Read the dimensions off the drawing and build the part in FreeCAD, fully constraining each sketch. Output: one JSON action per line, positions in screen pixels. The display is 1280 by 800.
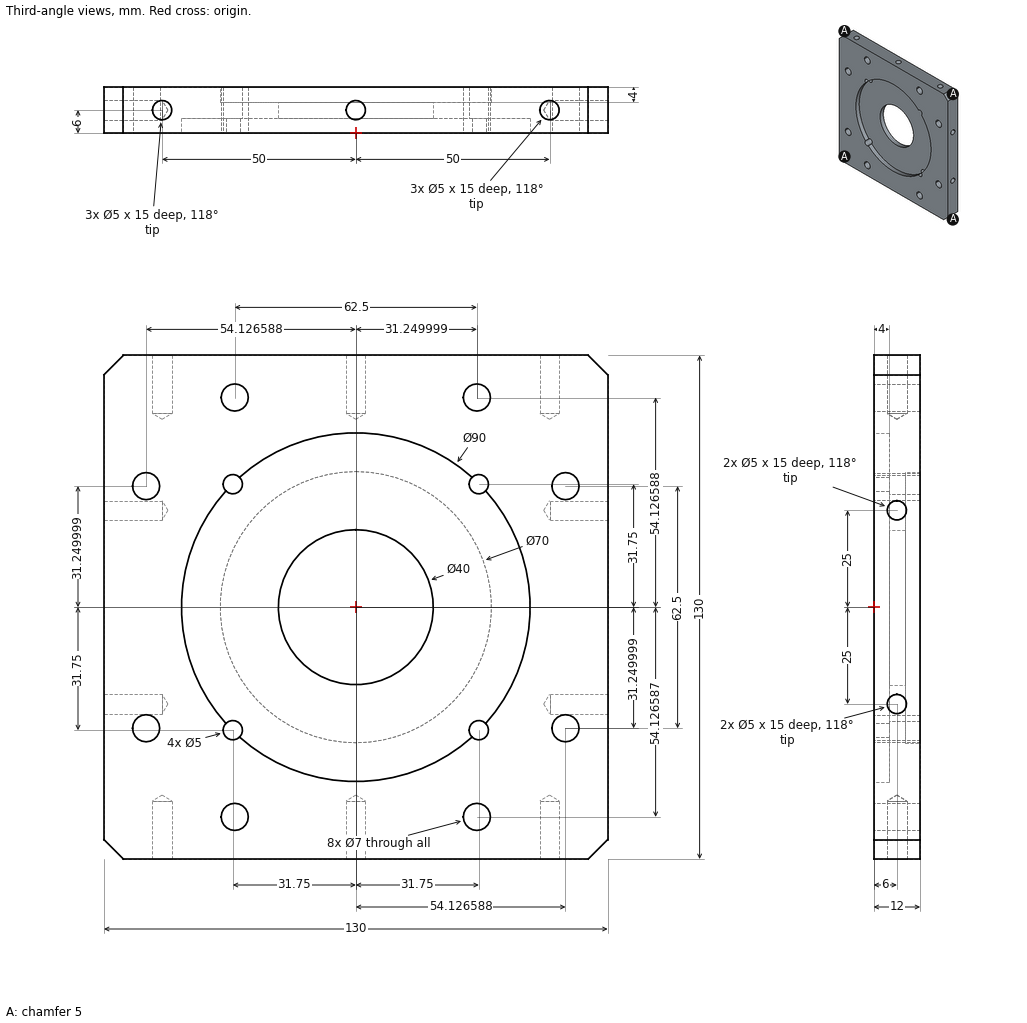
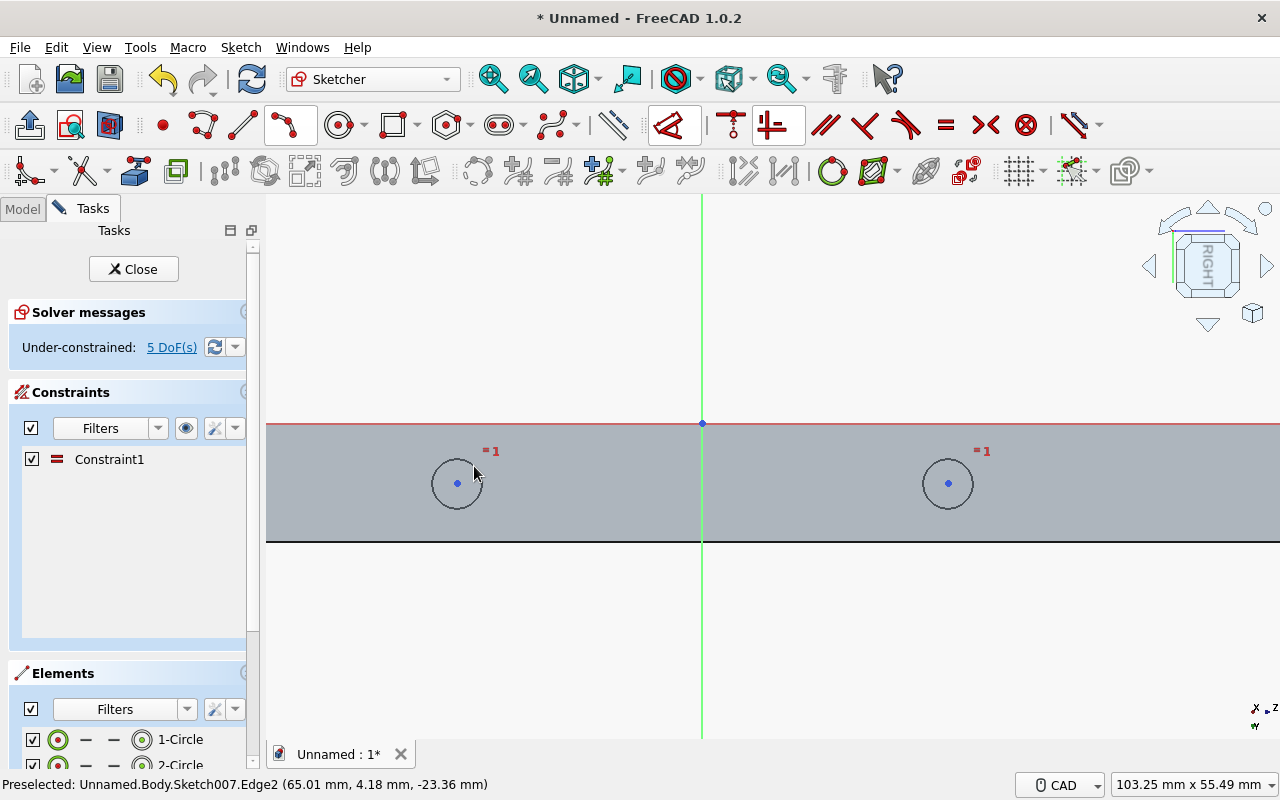
{"action": "left_click", "coordinate": [948, 484]}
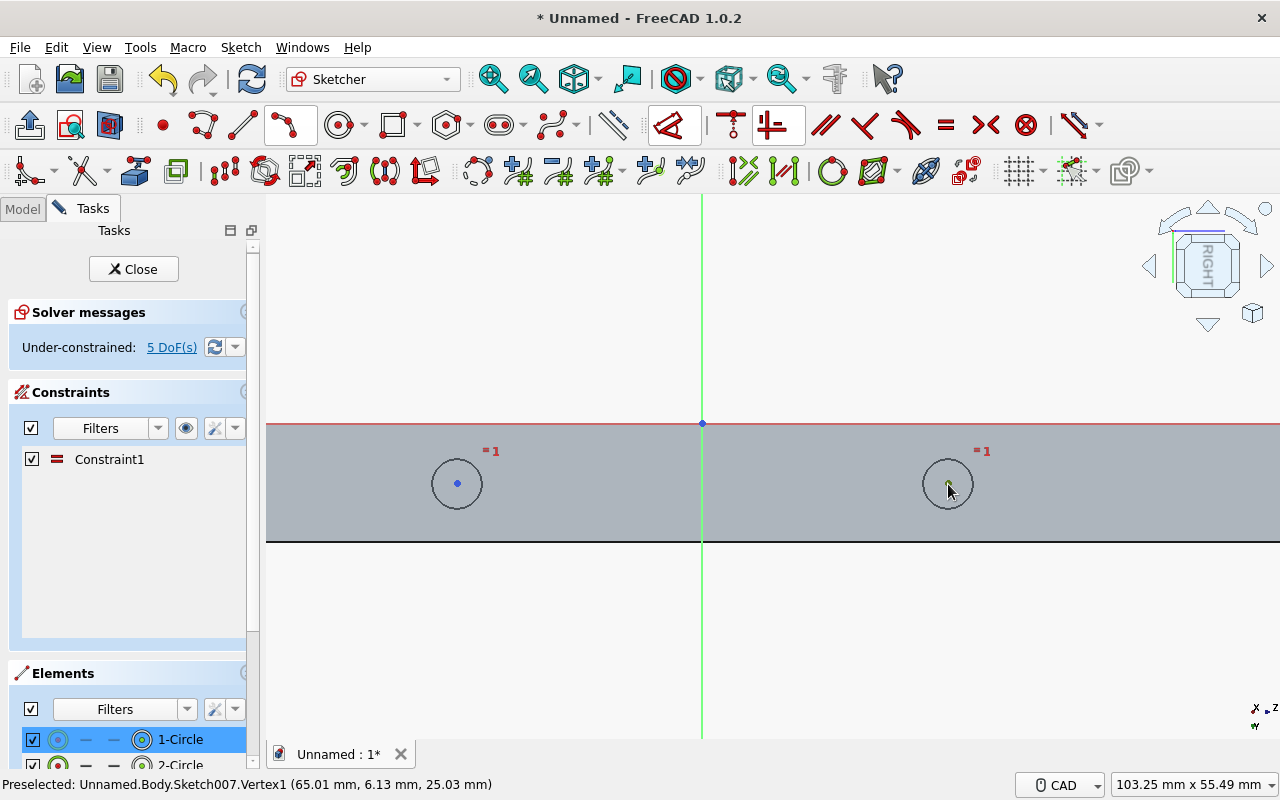
{"action": "left_click", "coordinate": [457, 484]}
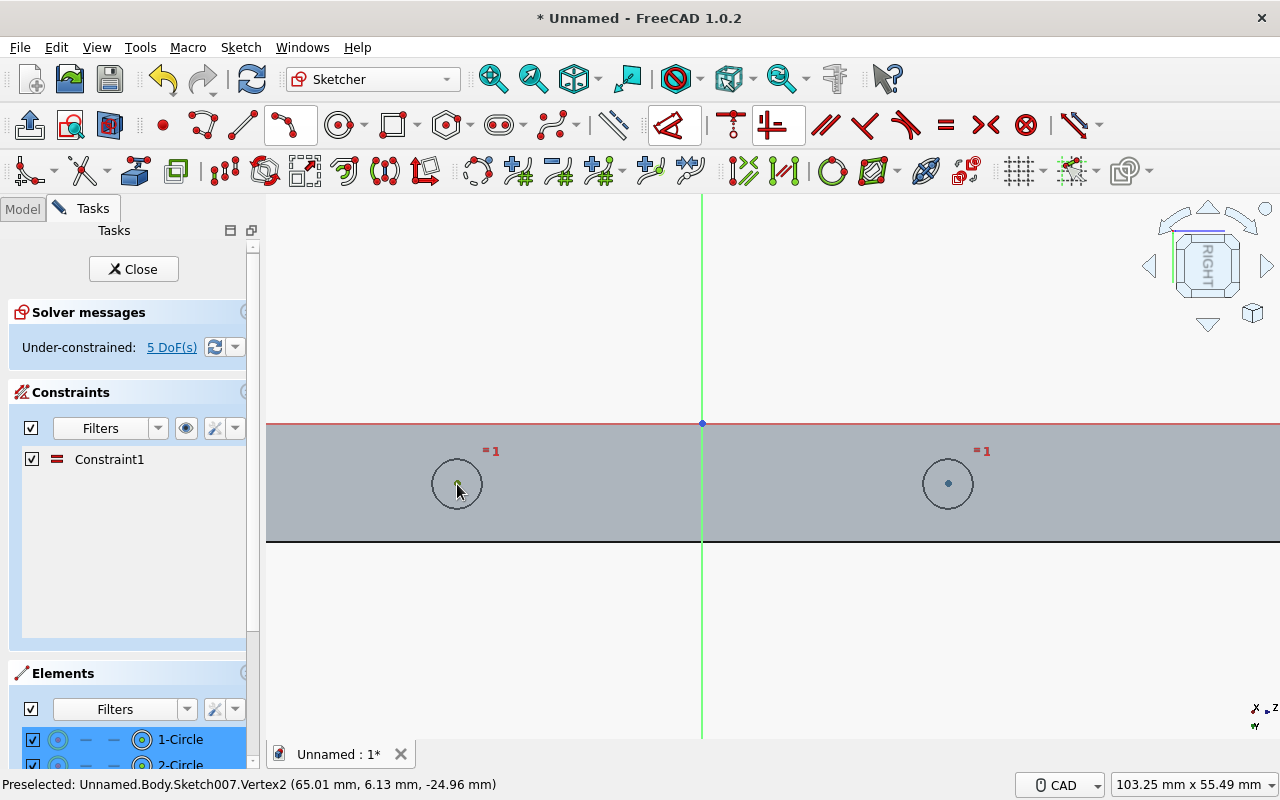
{"action": "left_click", "coordinate": [800, 126]}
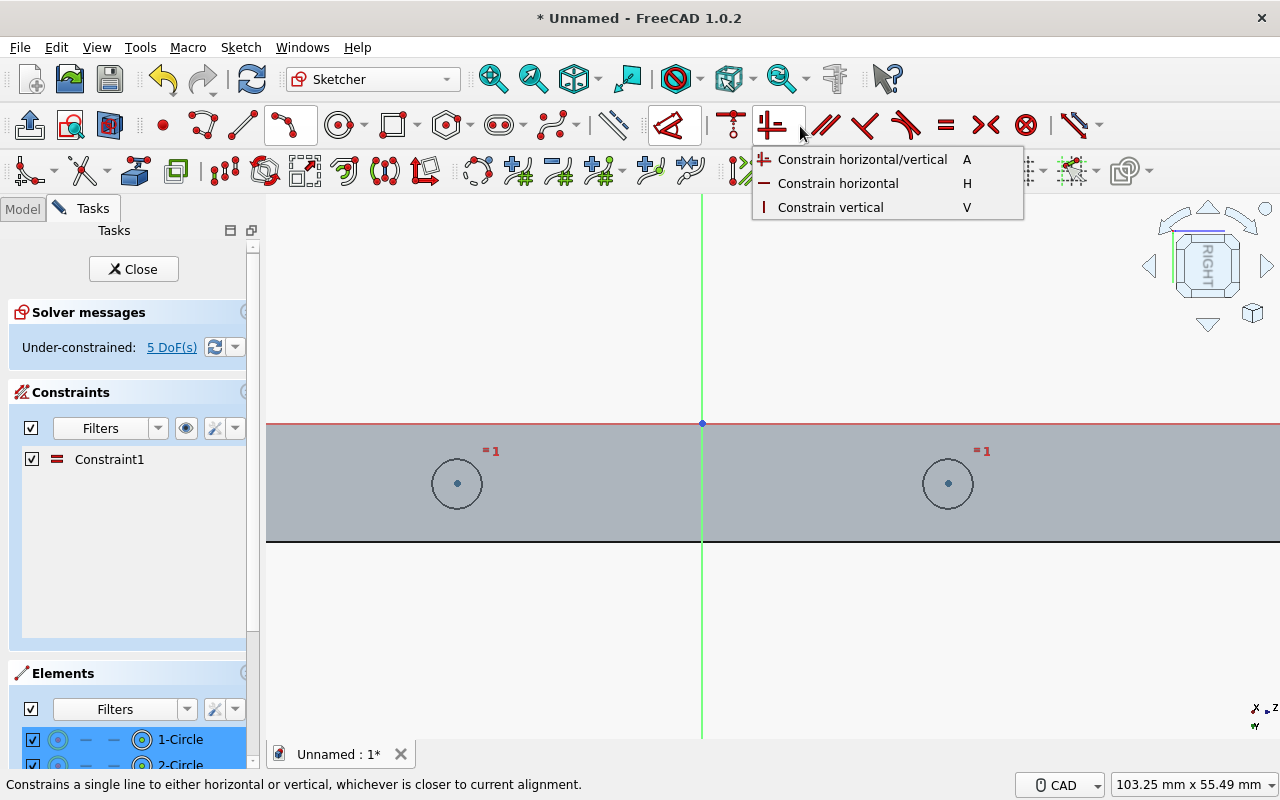
{"action": "left_click", "coordinate": [888, 183]}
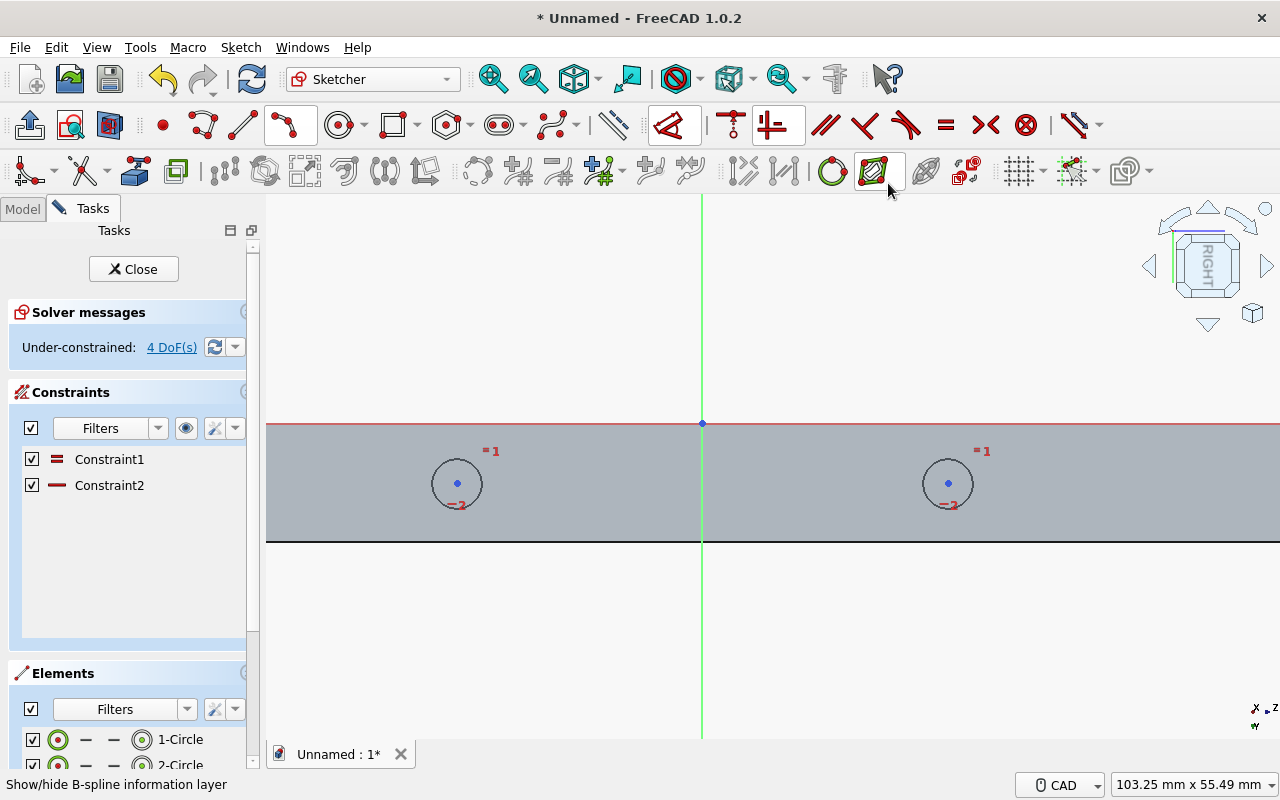
{"action": "left_click", "coordinate": [668, 126]}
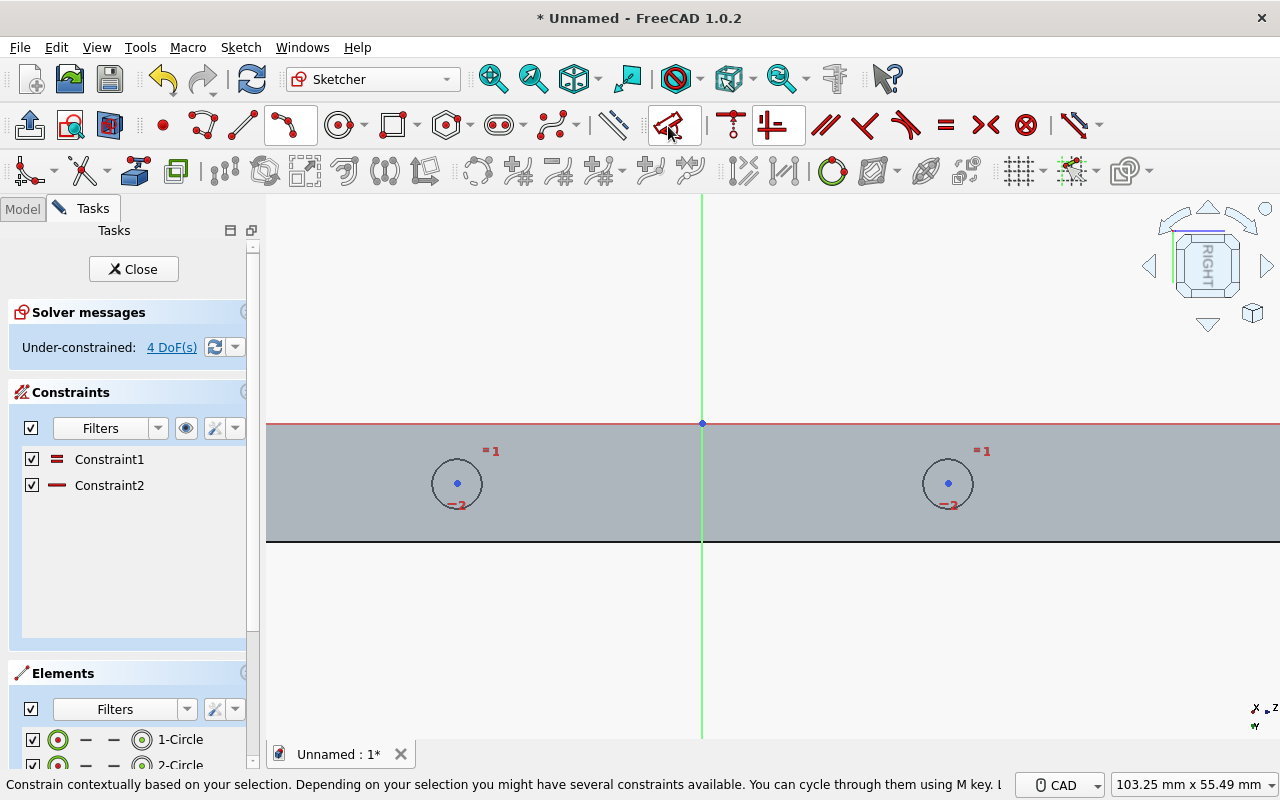
{"action": "left_click", "coordinate": [965, 466]}
{"action": "left_click", "coordinate": [987, 443]}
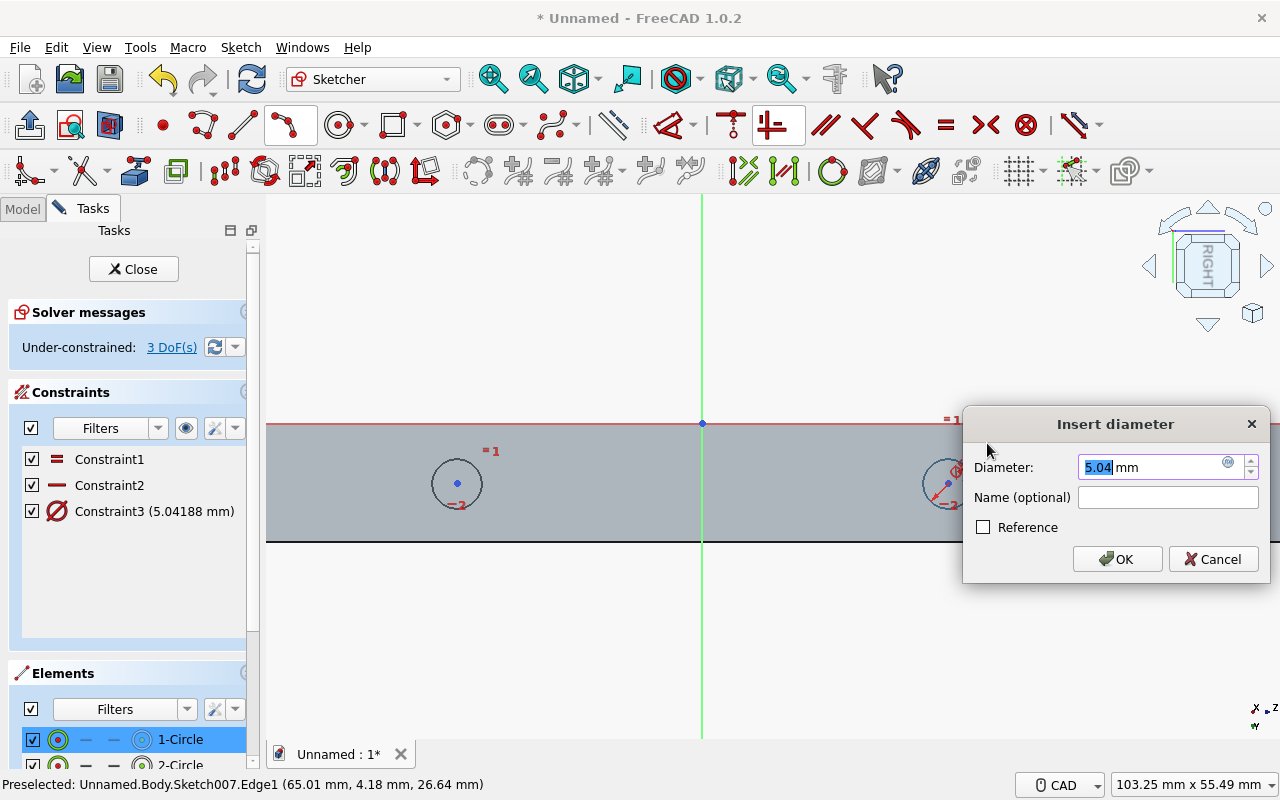
{"action": "type", "text": "5"}
{"action": "key", "text": "Return"}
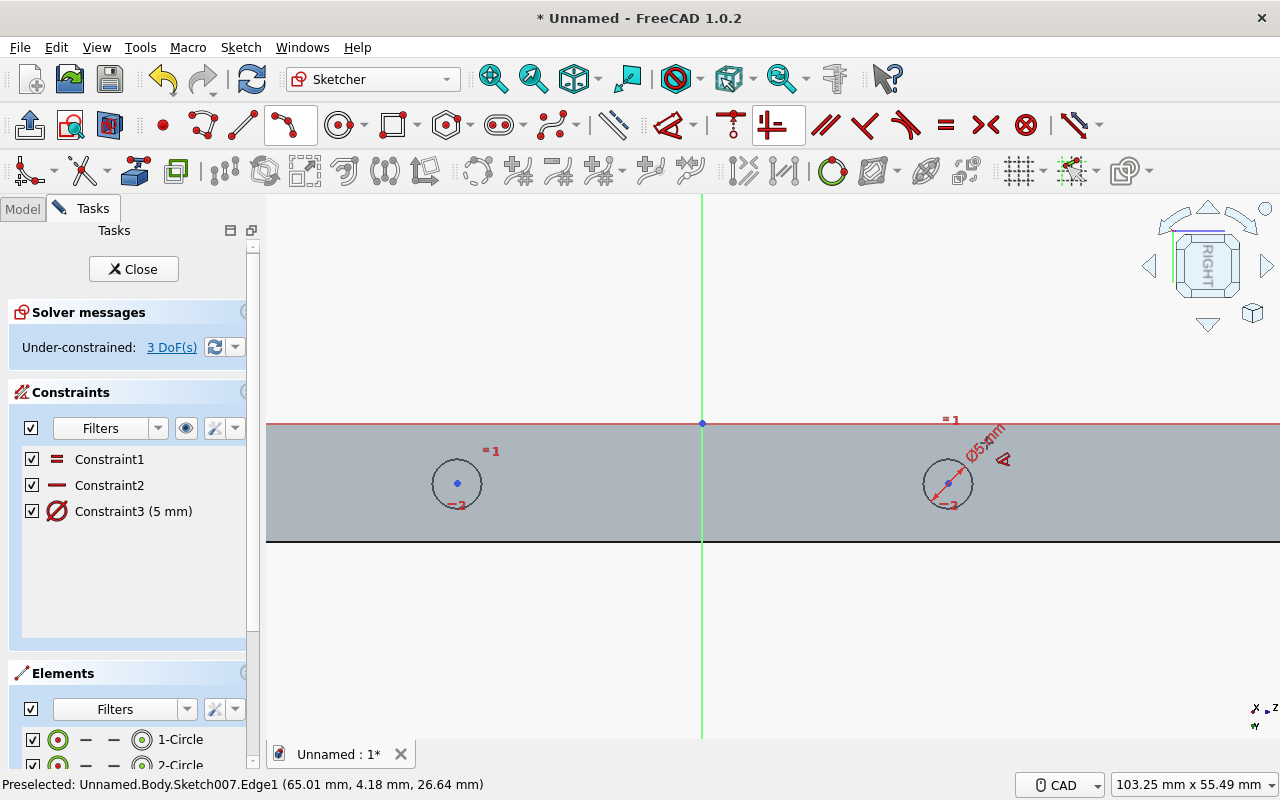
{"action": "left_click", "coordinate": [948, 484]}
{"action": "left_click", "coordinate": [982, 468]}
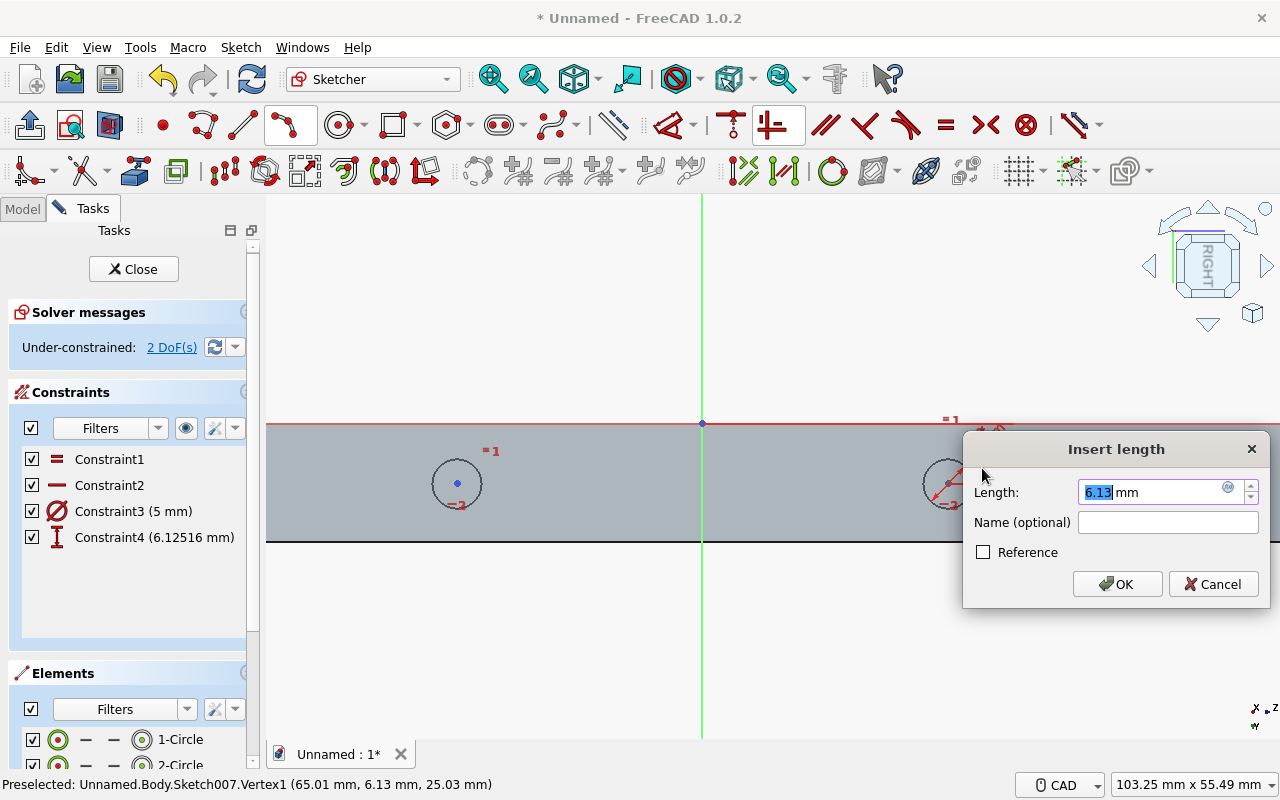
{"action": "type", "text": "6"}
{"action": "key", "text": "Return"}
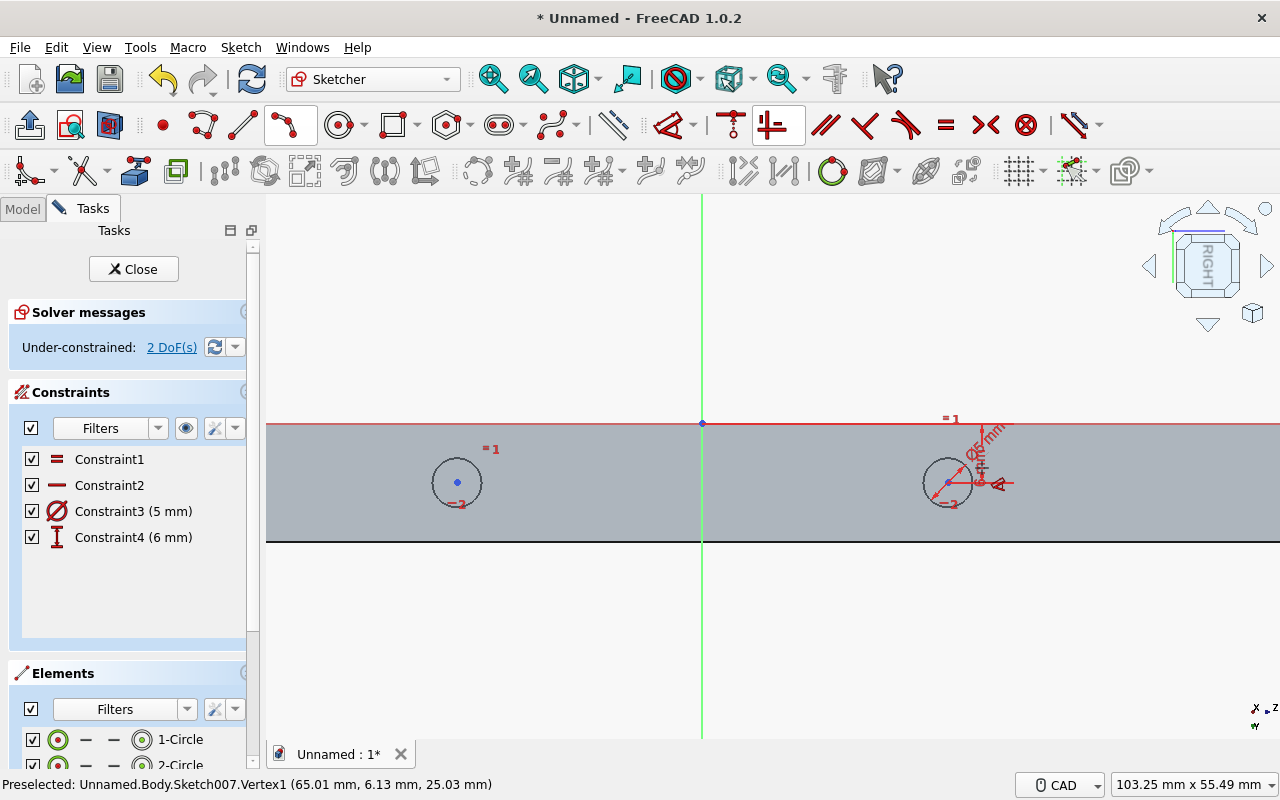
{"action": "left_click", "coordinate": [948, 483]}
{"action": "left_click", "coordinate": [825, 390]}